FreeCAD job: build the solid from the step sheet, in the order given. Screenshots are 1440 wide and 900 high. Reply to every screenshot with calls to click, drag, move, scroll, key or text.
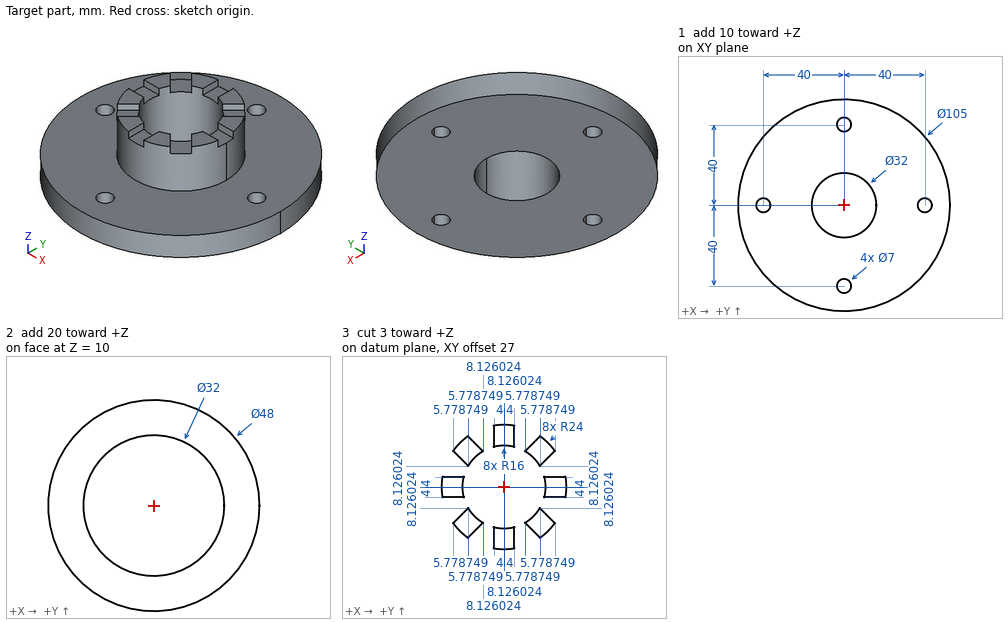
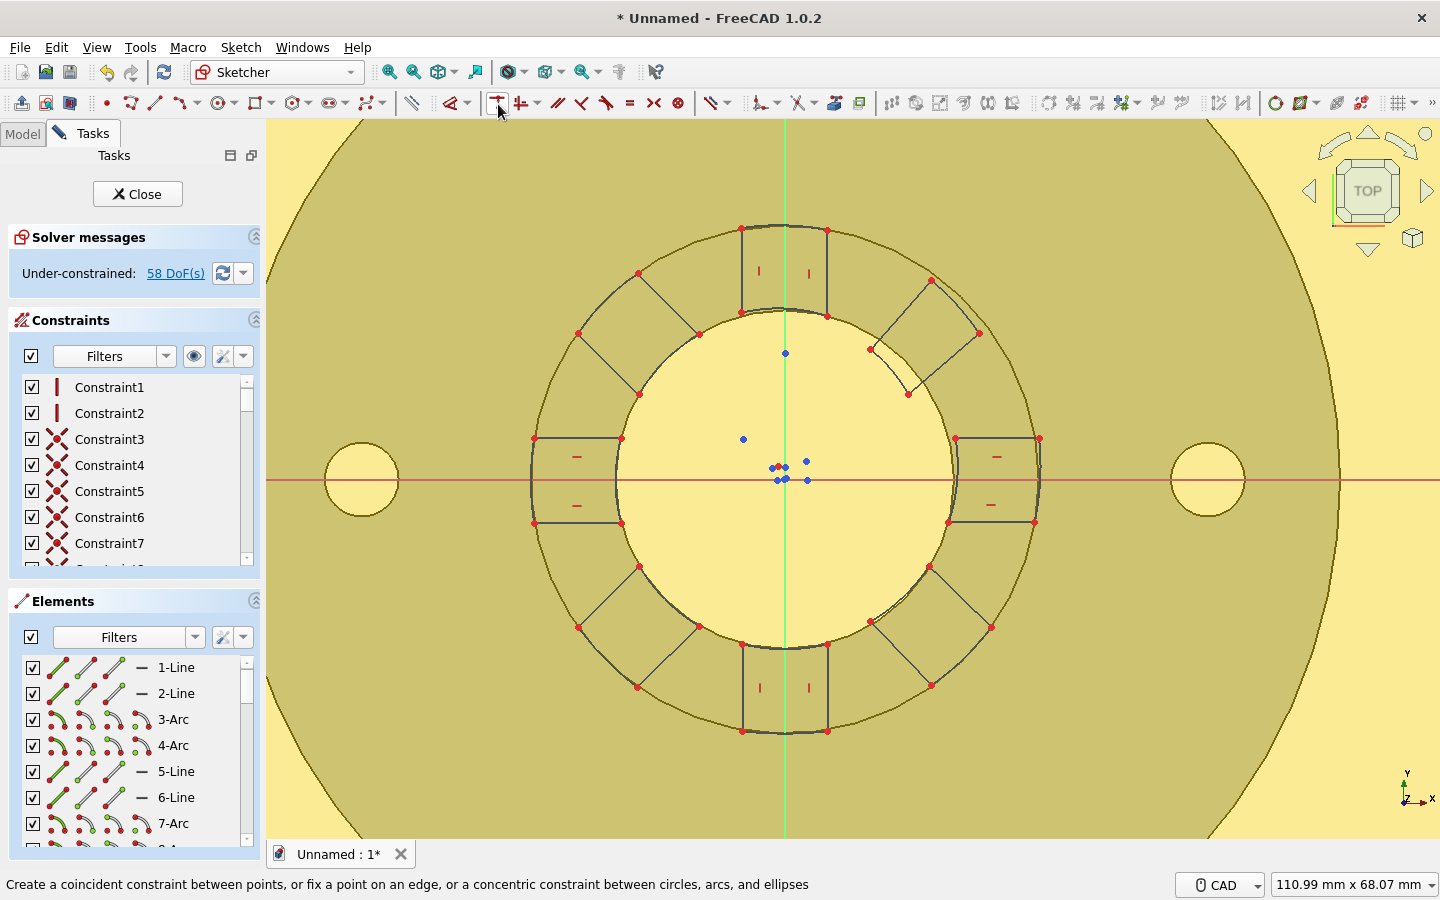
click(802, 310)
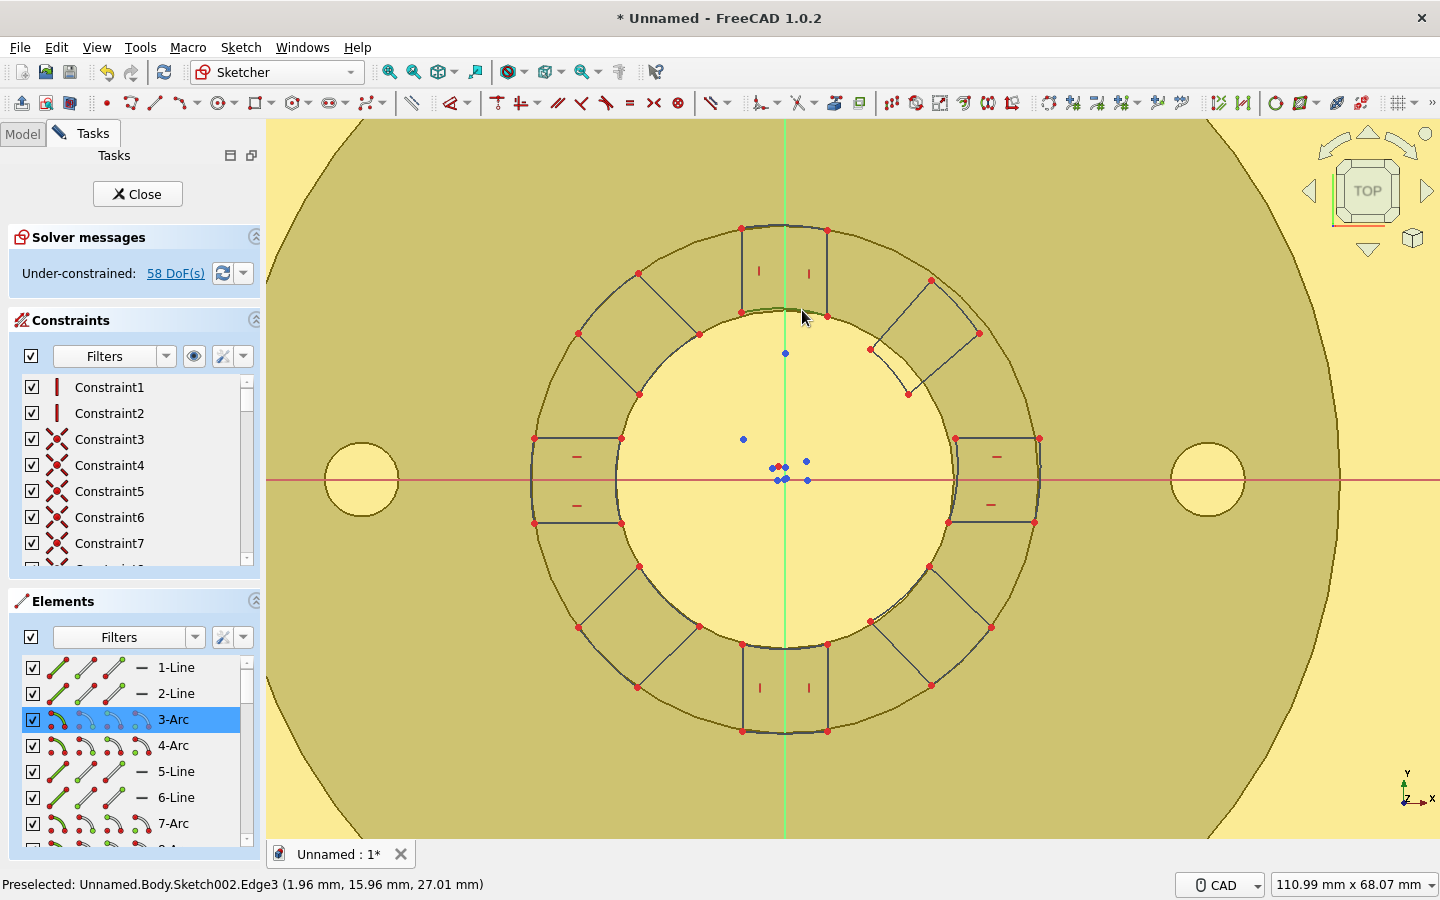
click(768, 648)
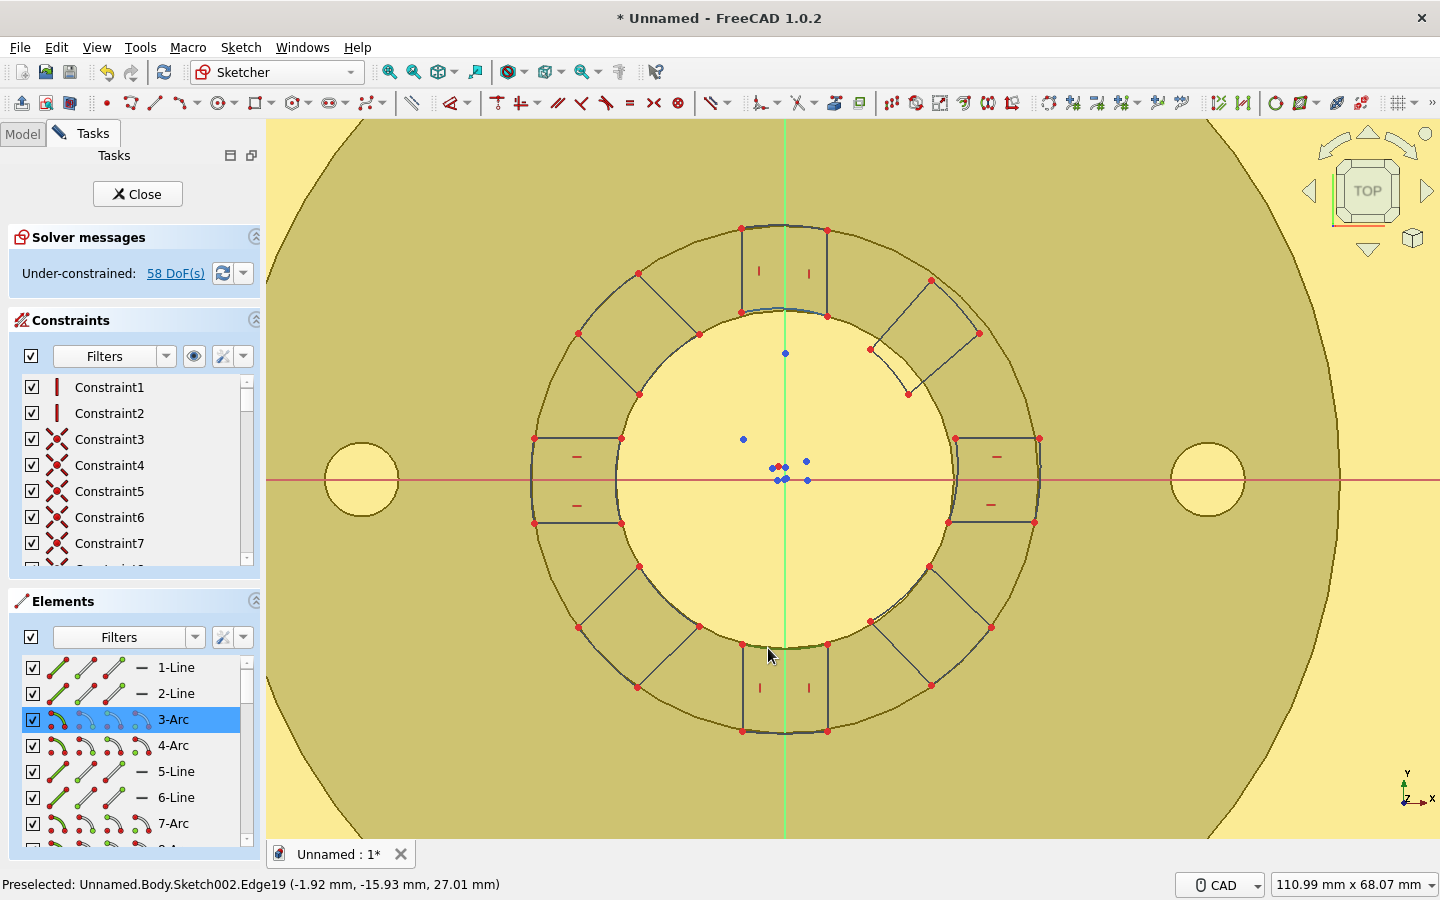
click(498, 104)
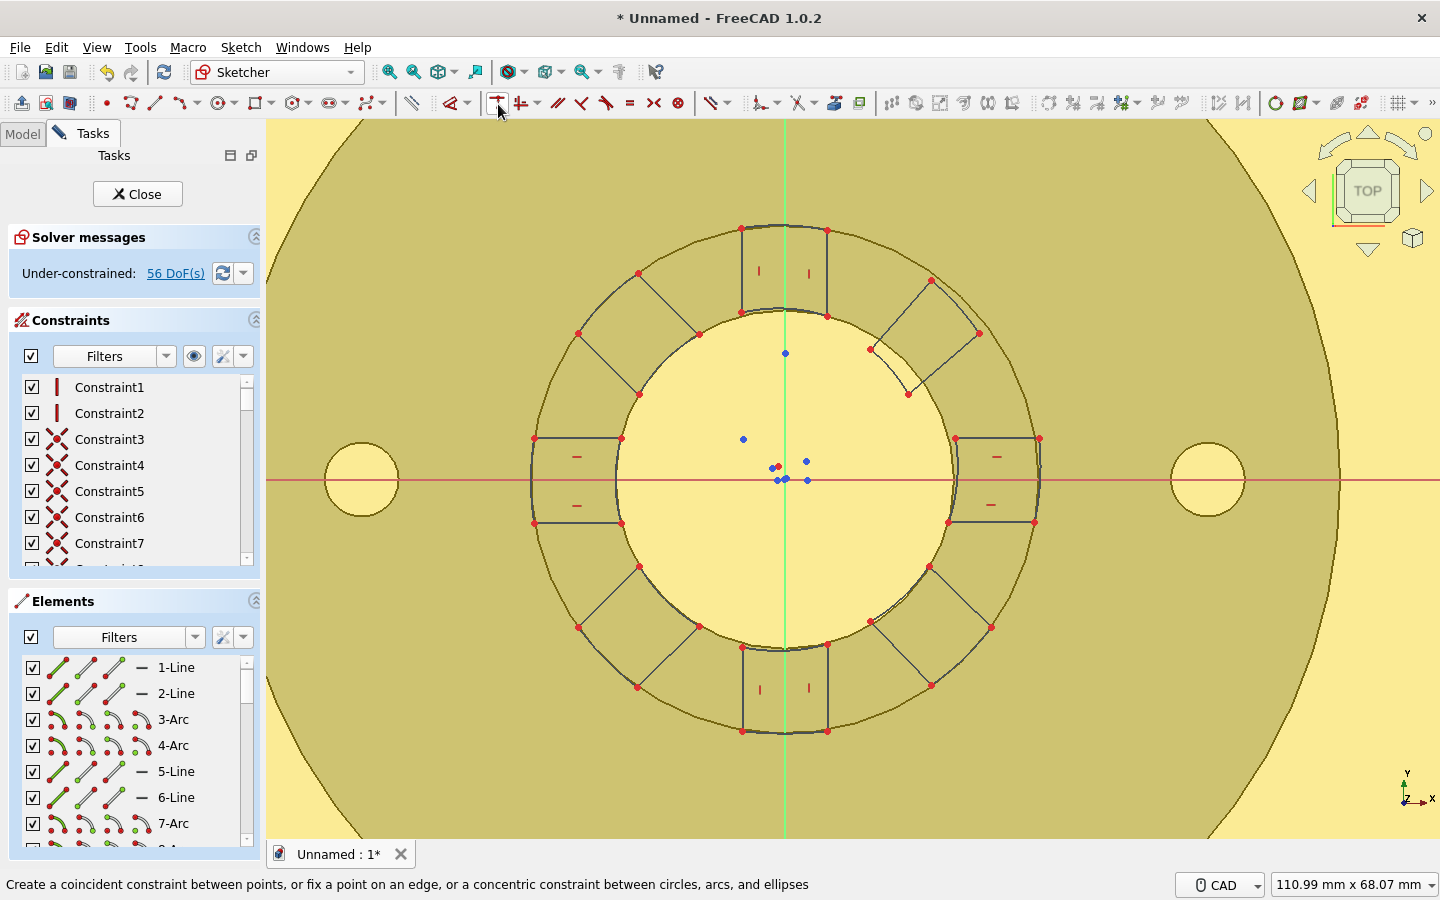
click(802, 310)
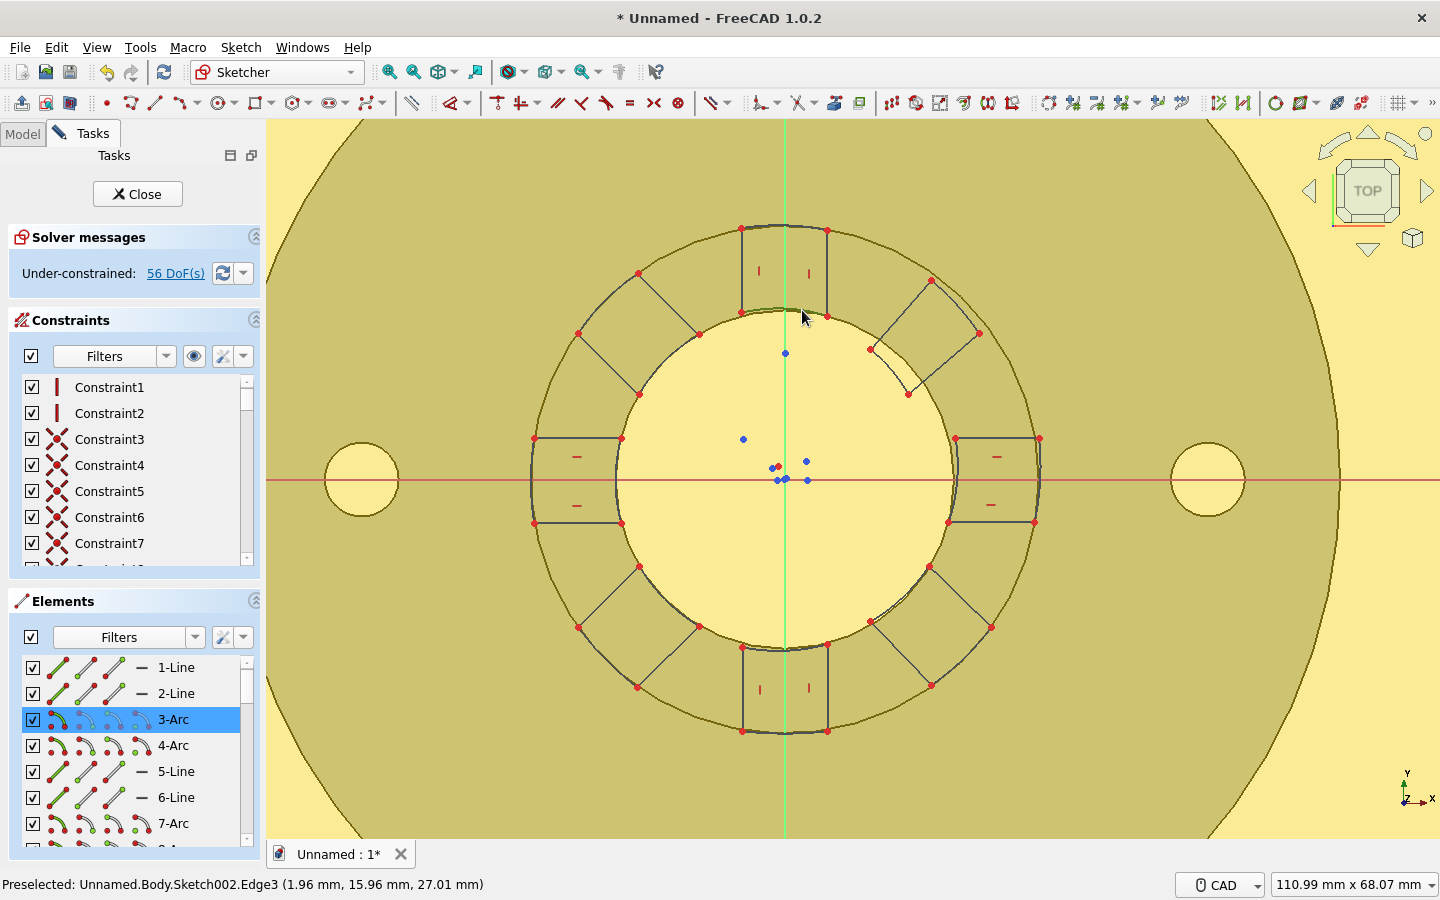
click(768, 733)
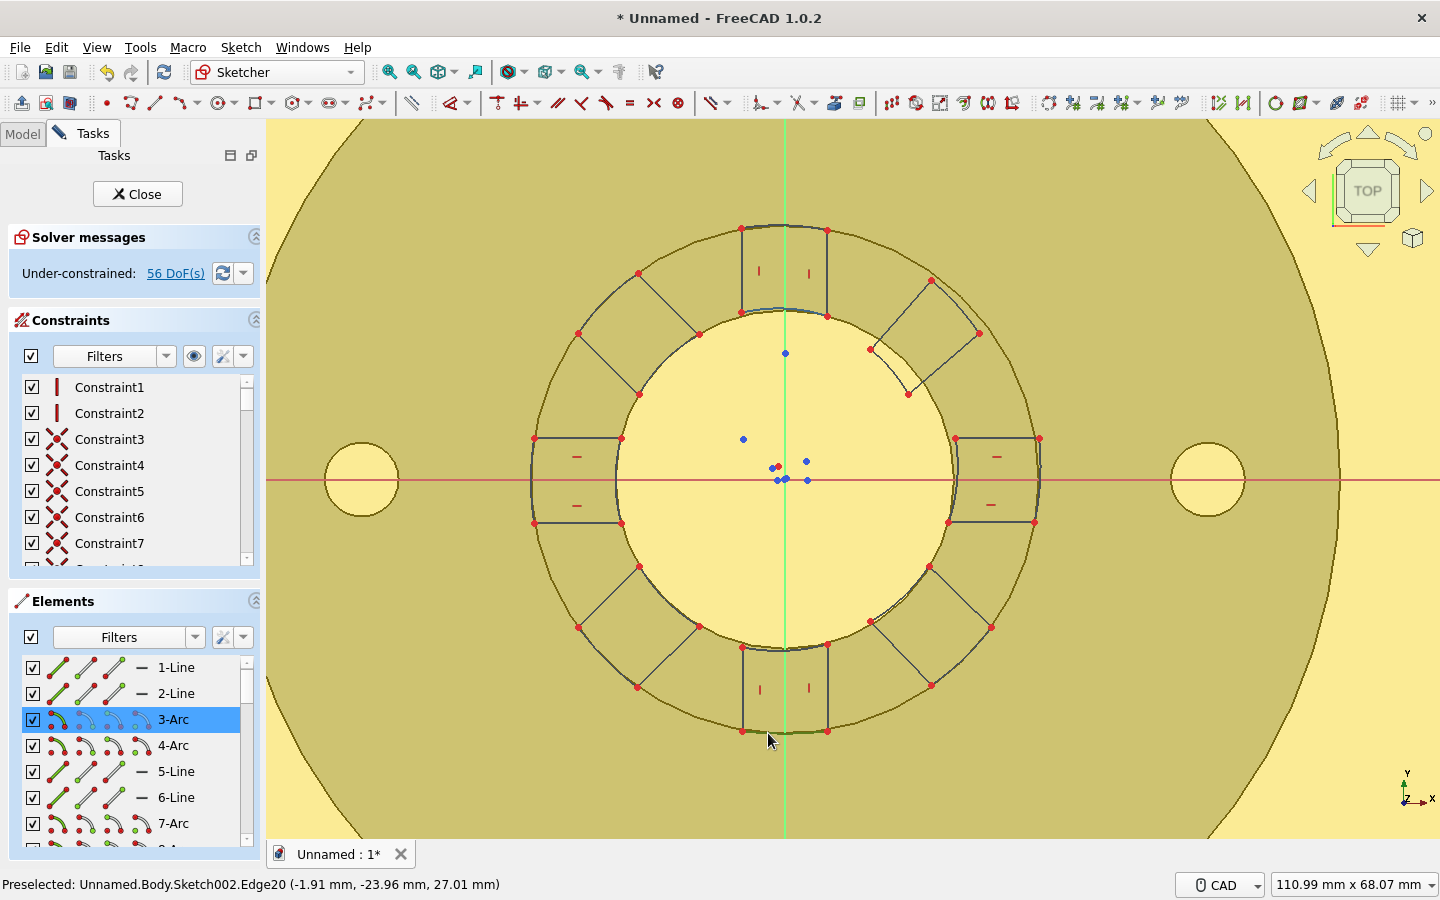
click(498, 104)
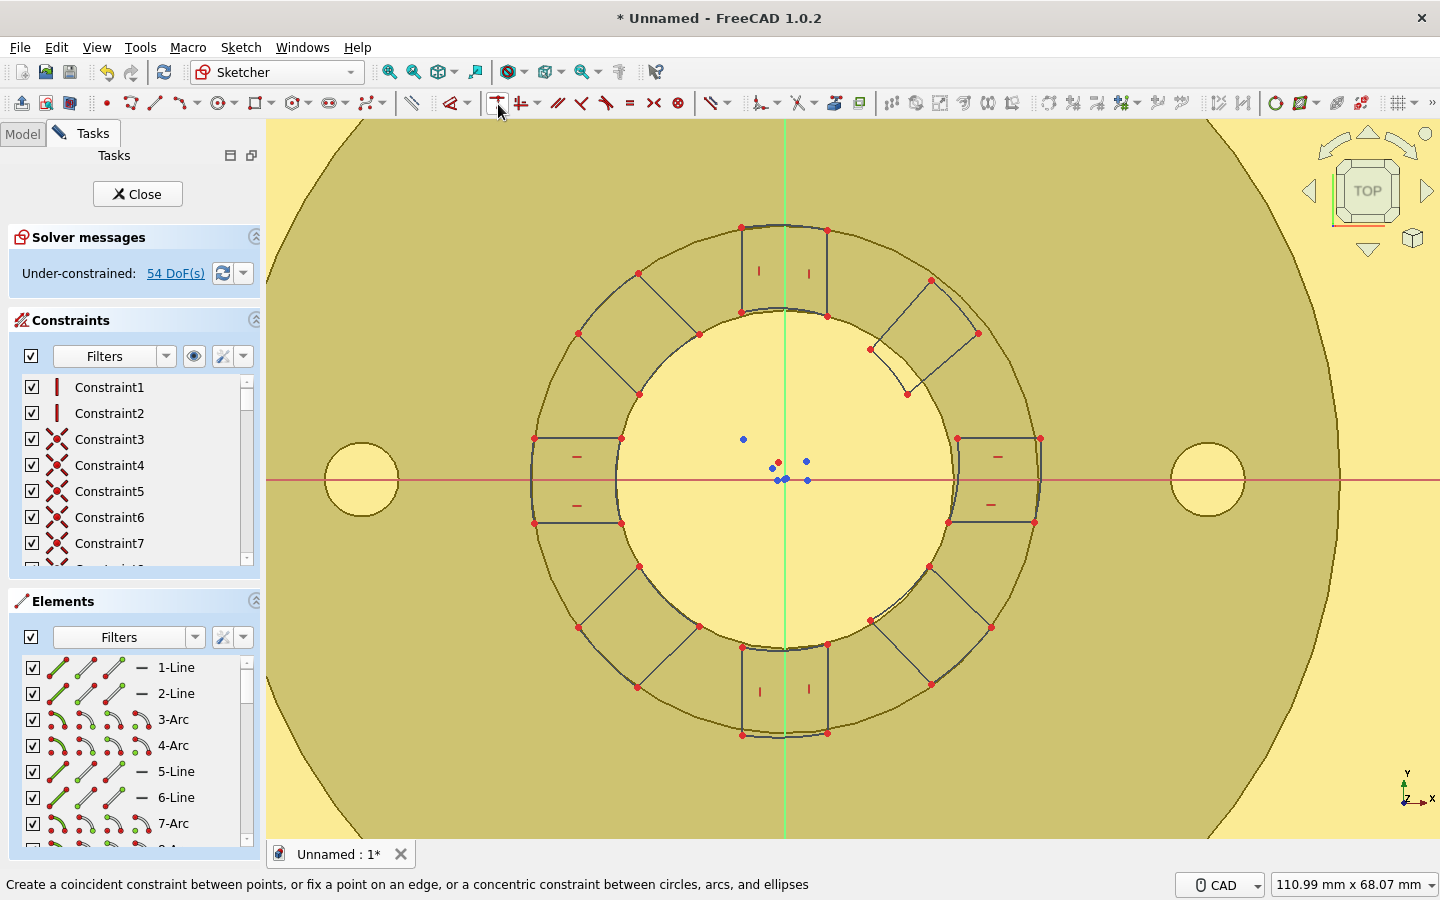
click(802, 310)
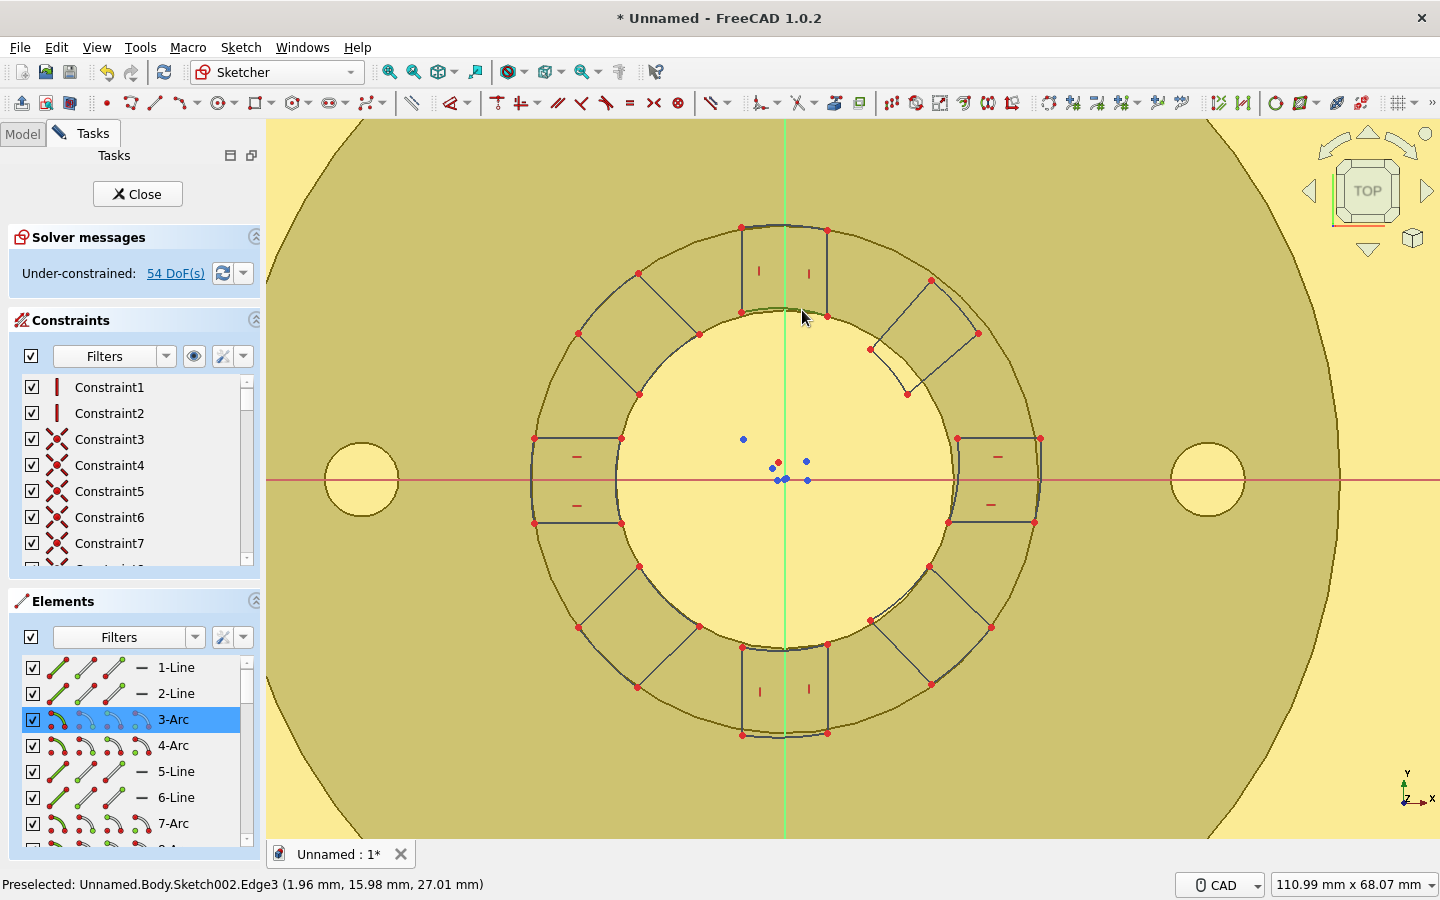
click(654, 587)